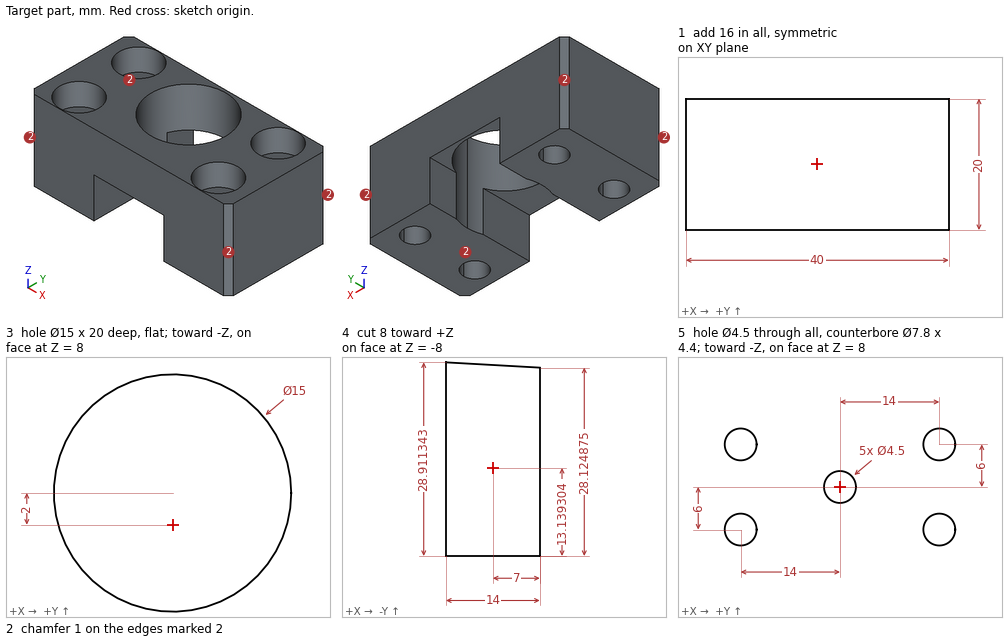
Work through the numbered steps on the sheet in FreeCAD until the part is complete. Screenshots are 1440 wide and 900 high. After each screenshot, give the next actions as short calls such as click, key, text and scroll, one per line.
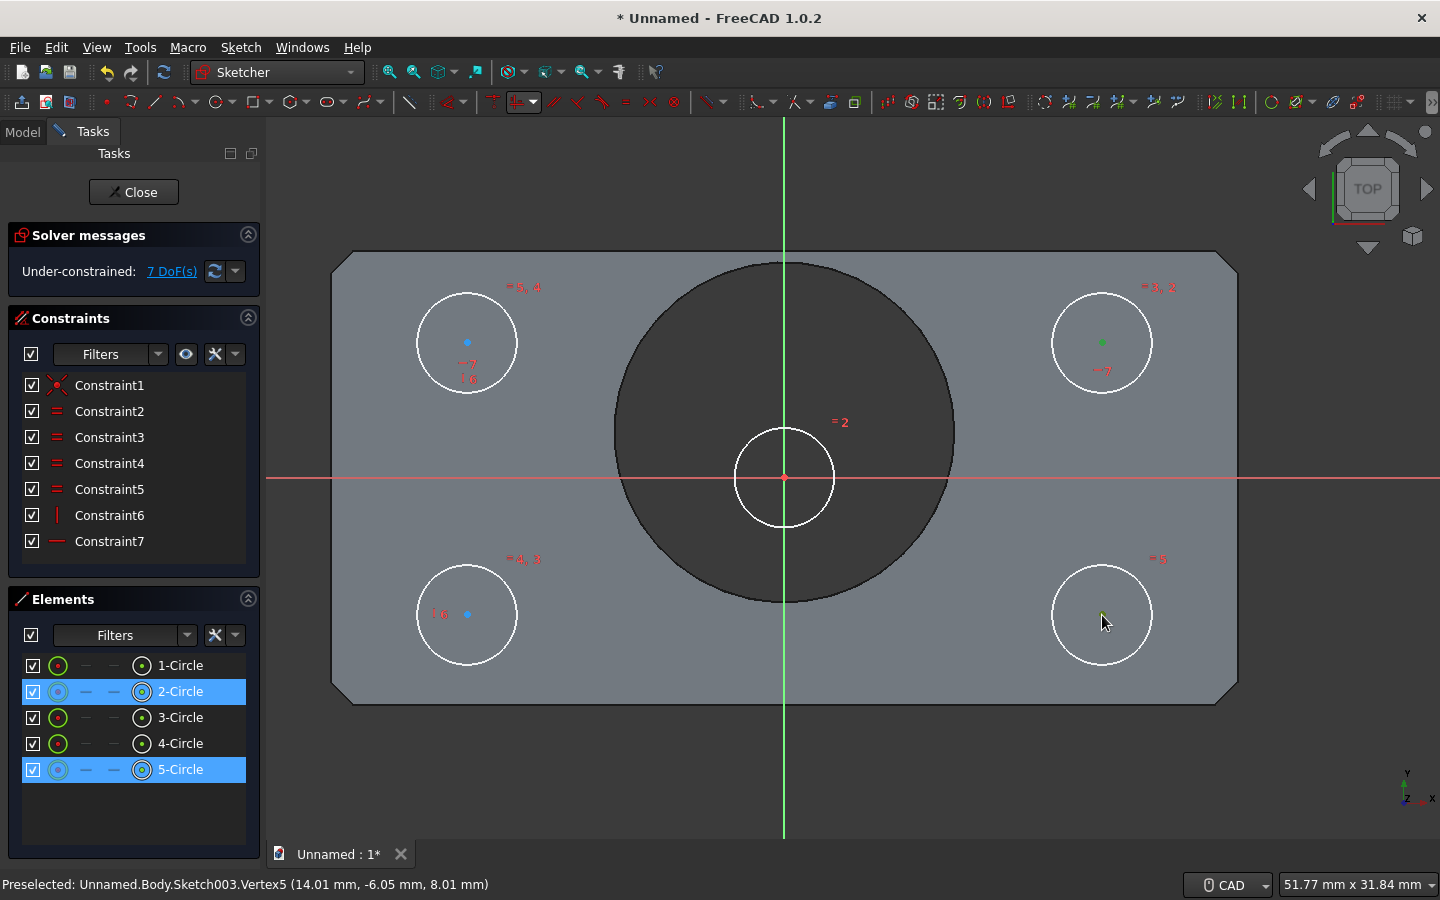
key(v)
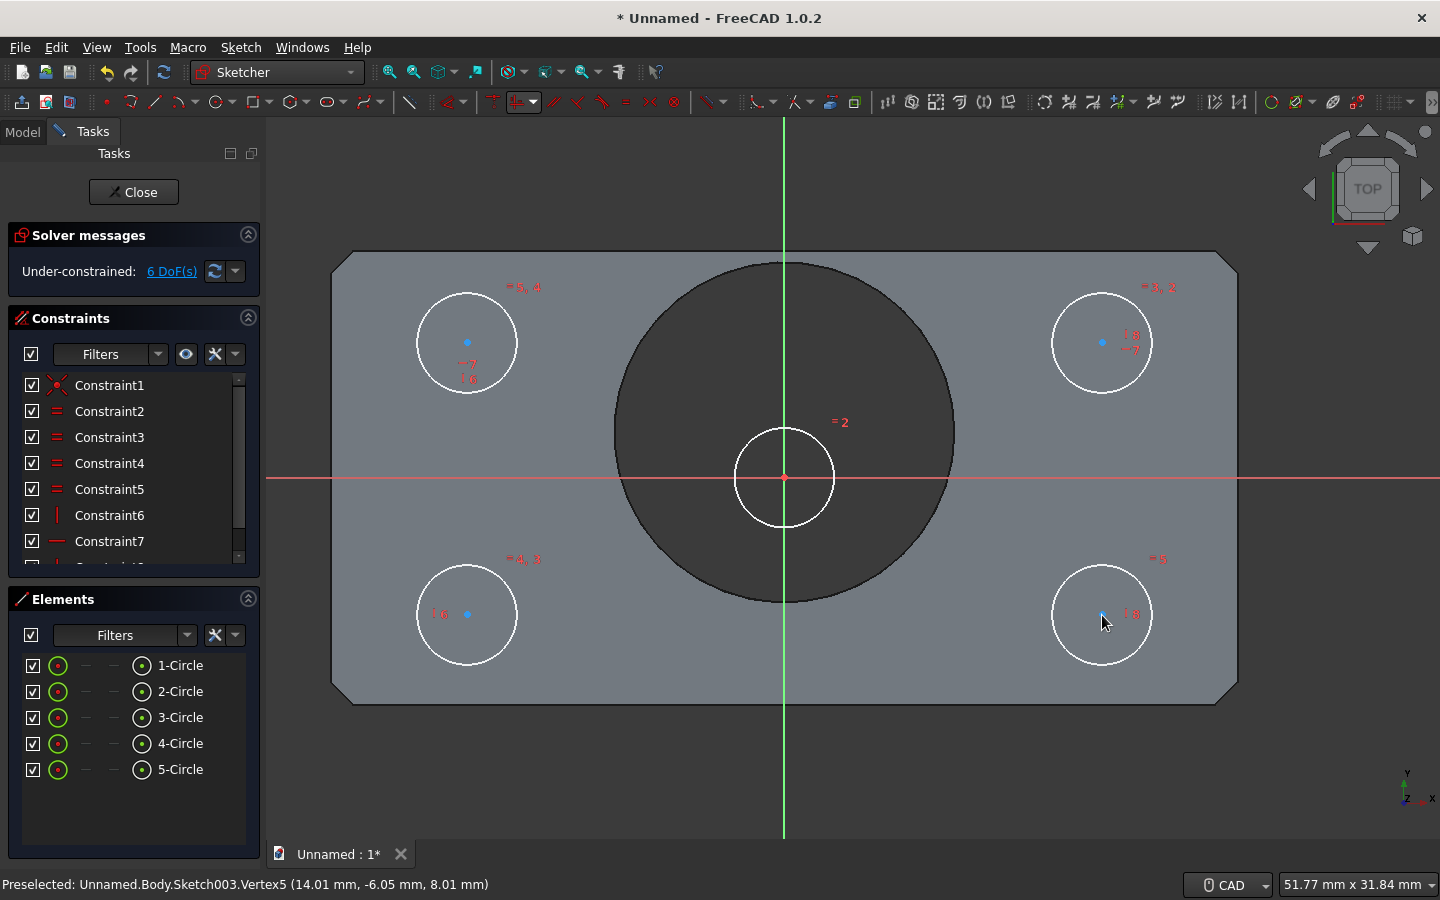
click(467, 615)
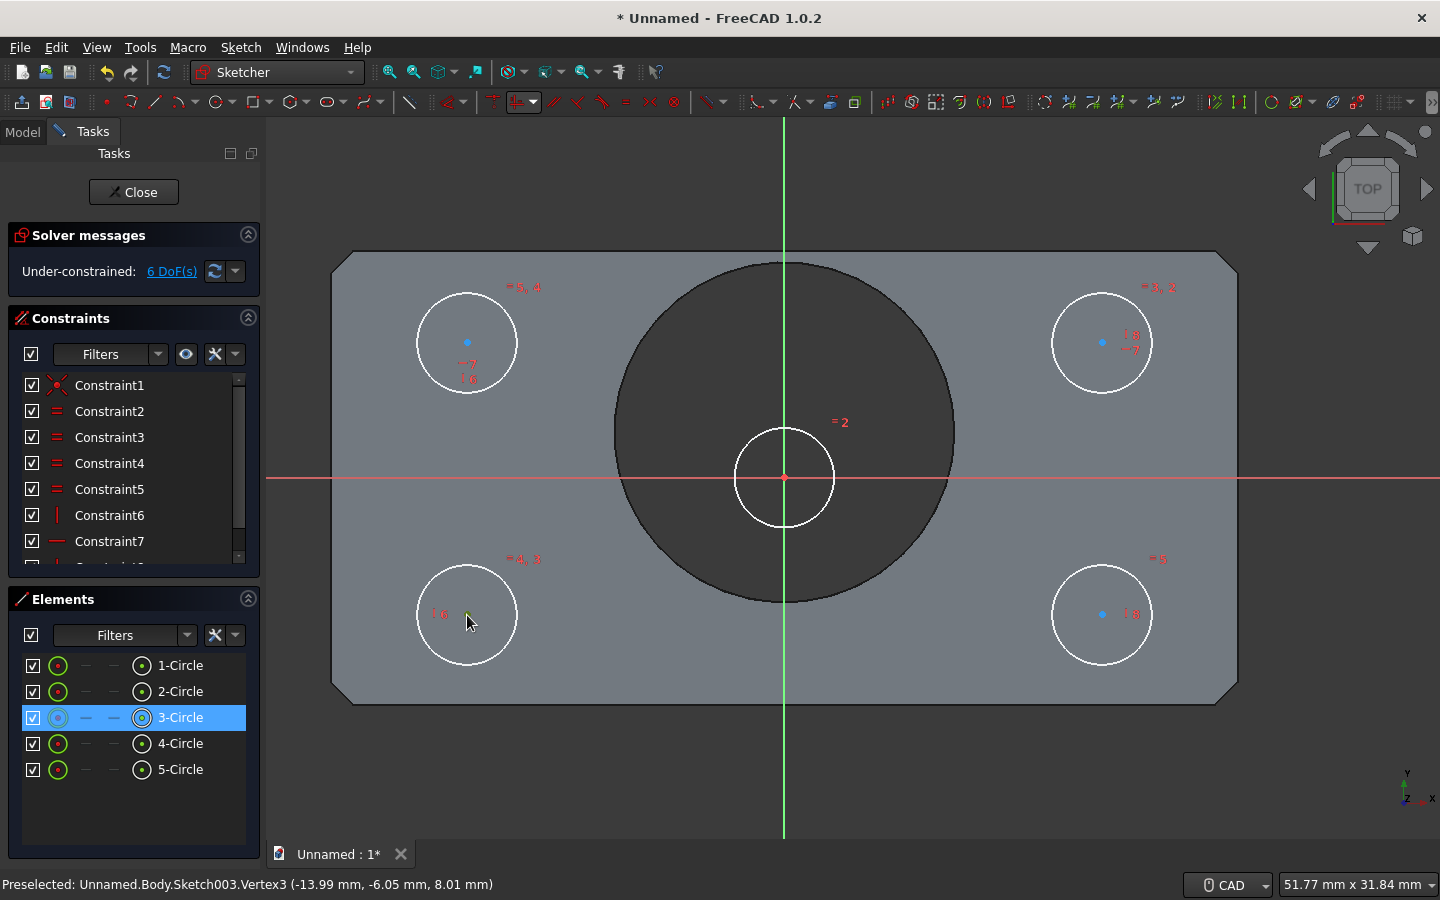
click(1102, 615)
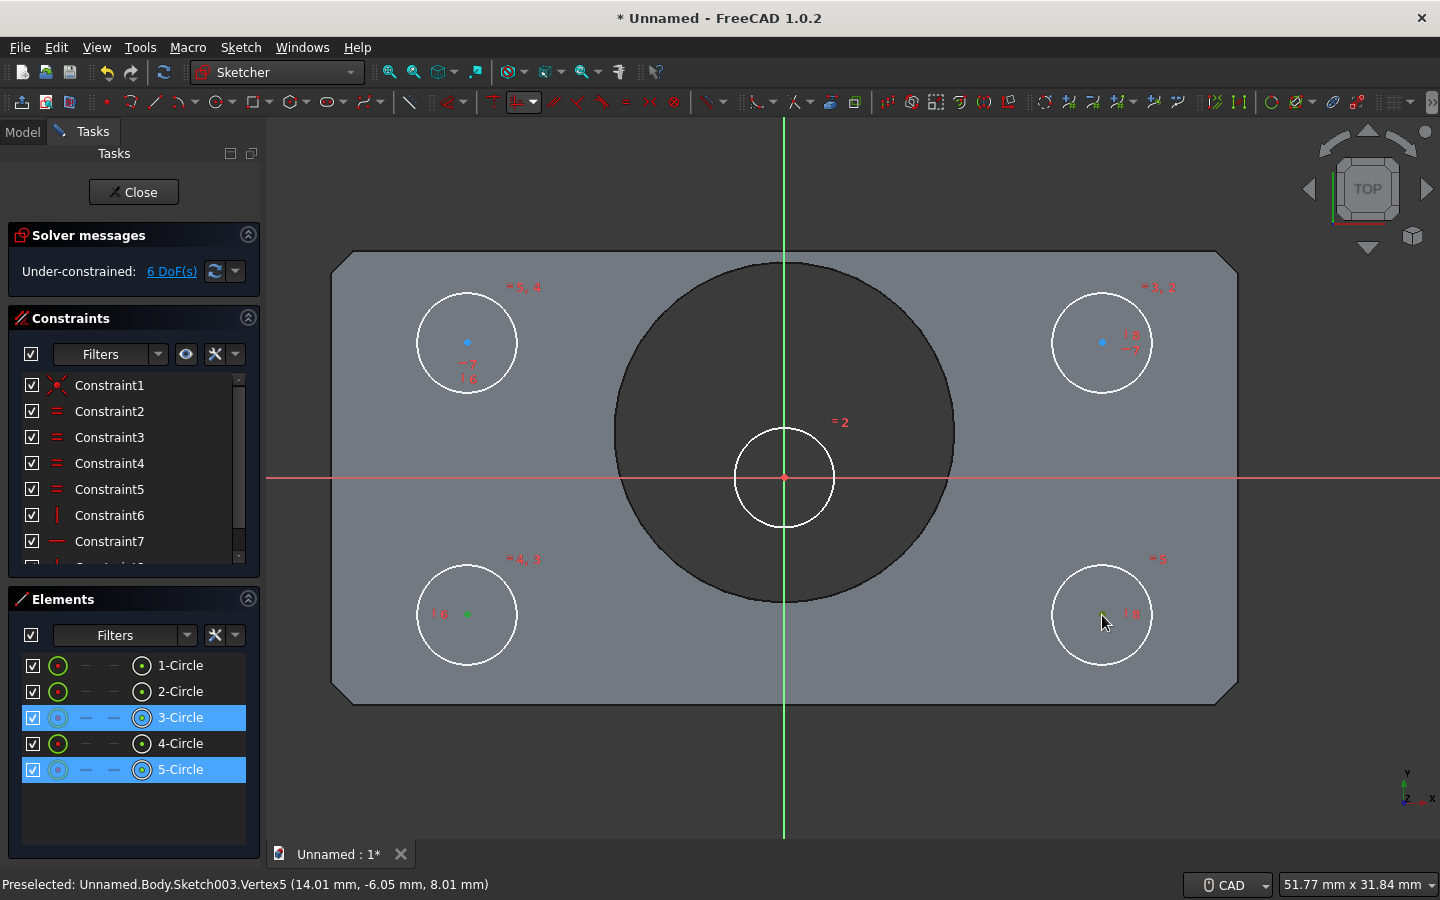
key(h)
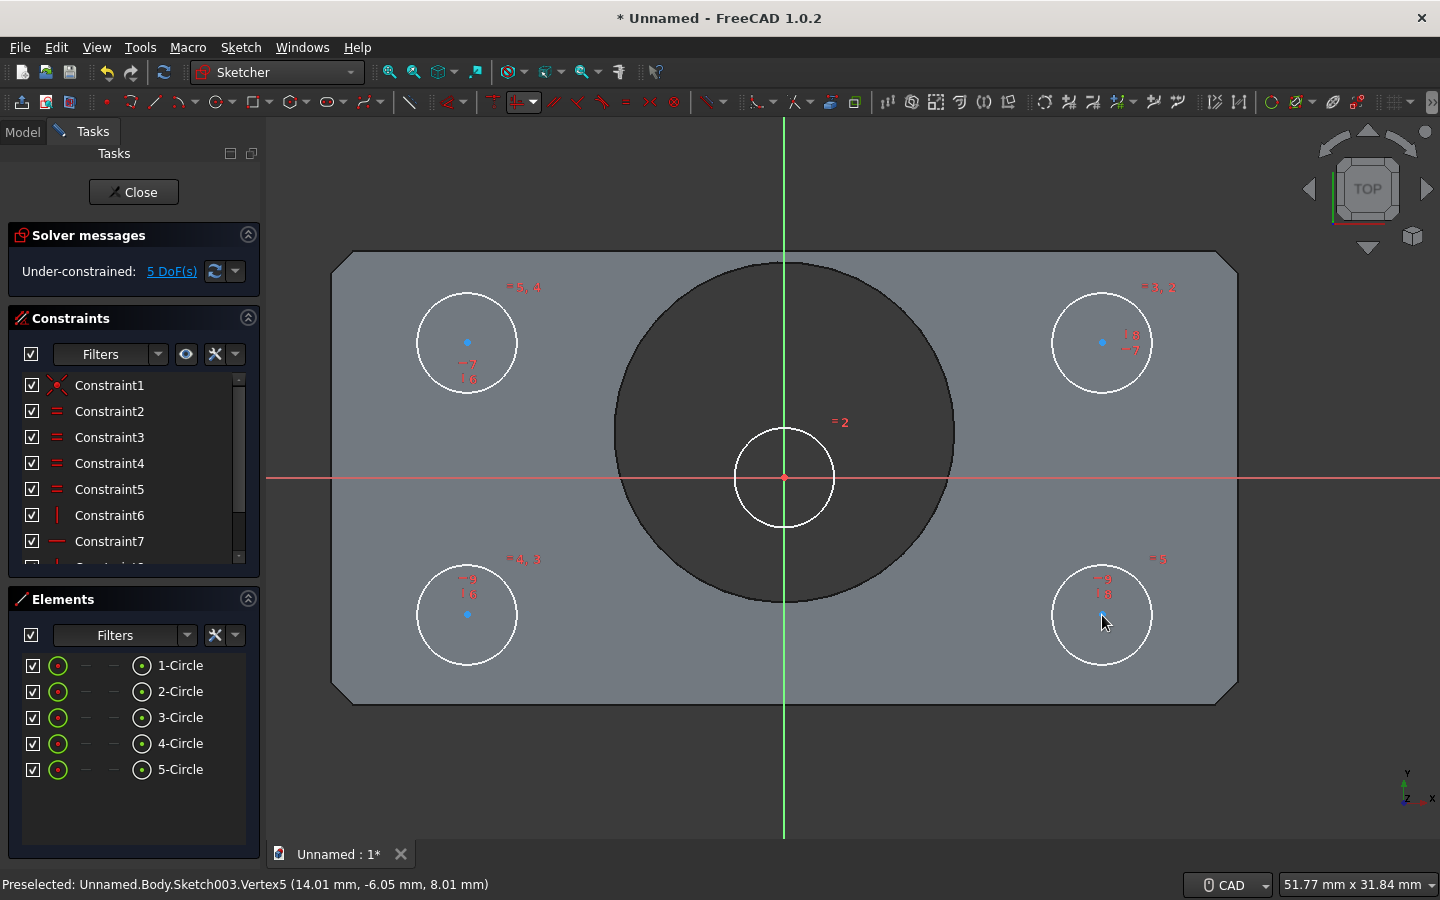
key(d)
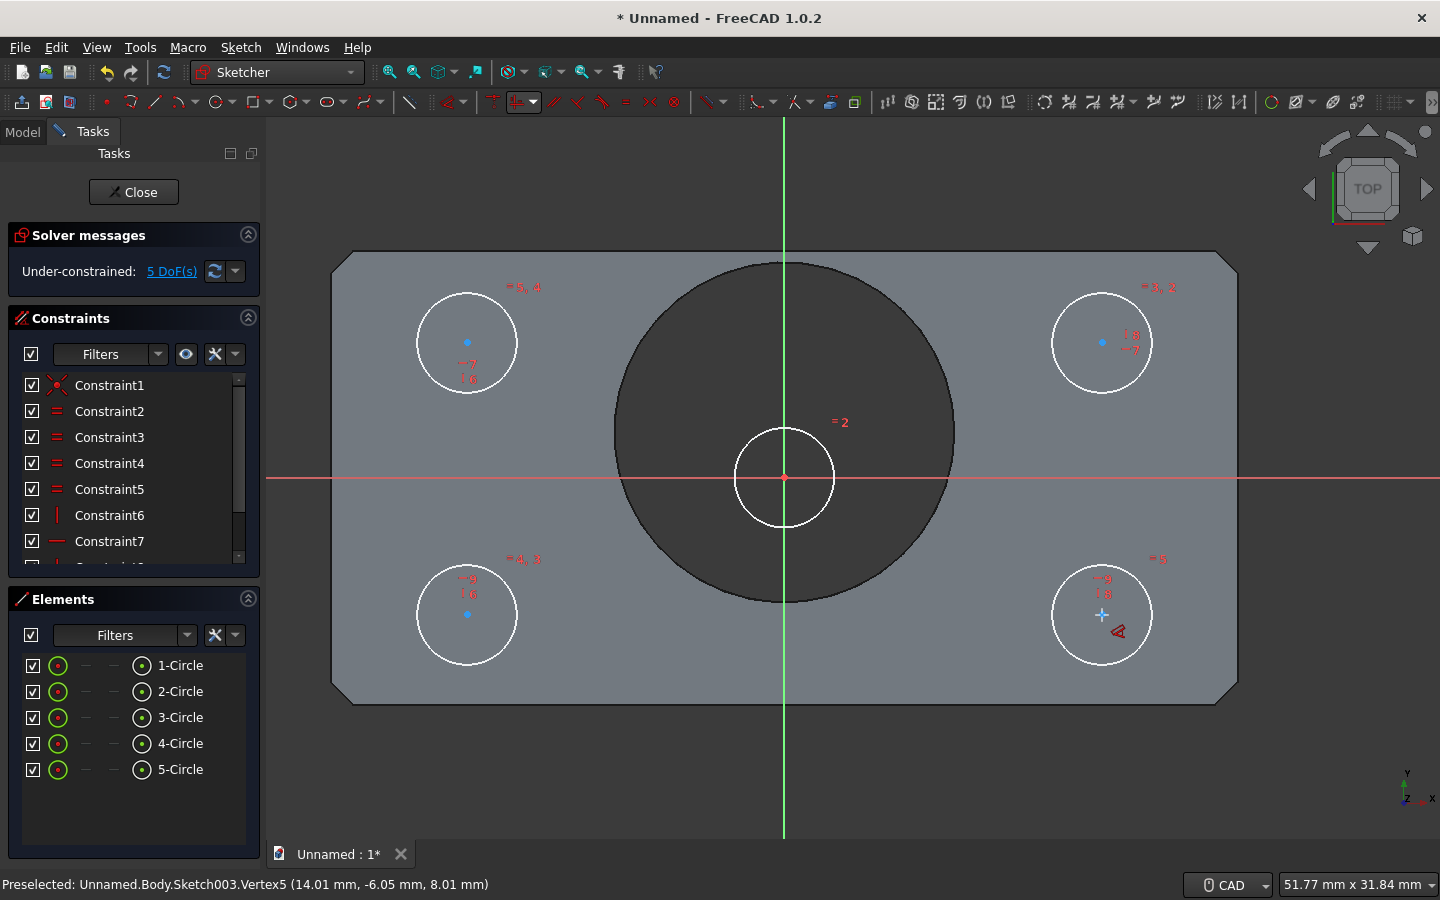
click(819, 442)
click(841, 419)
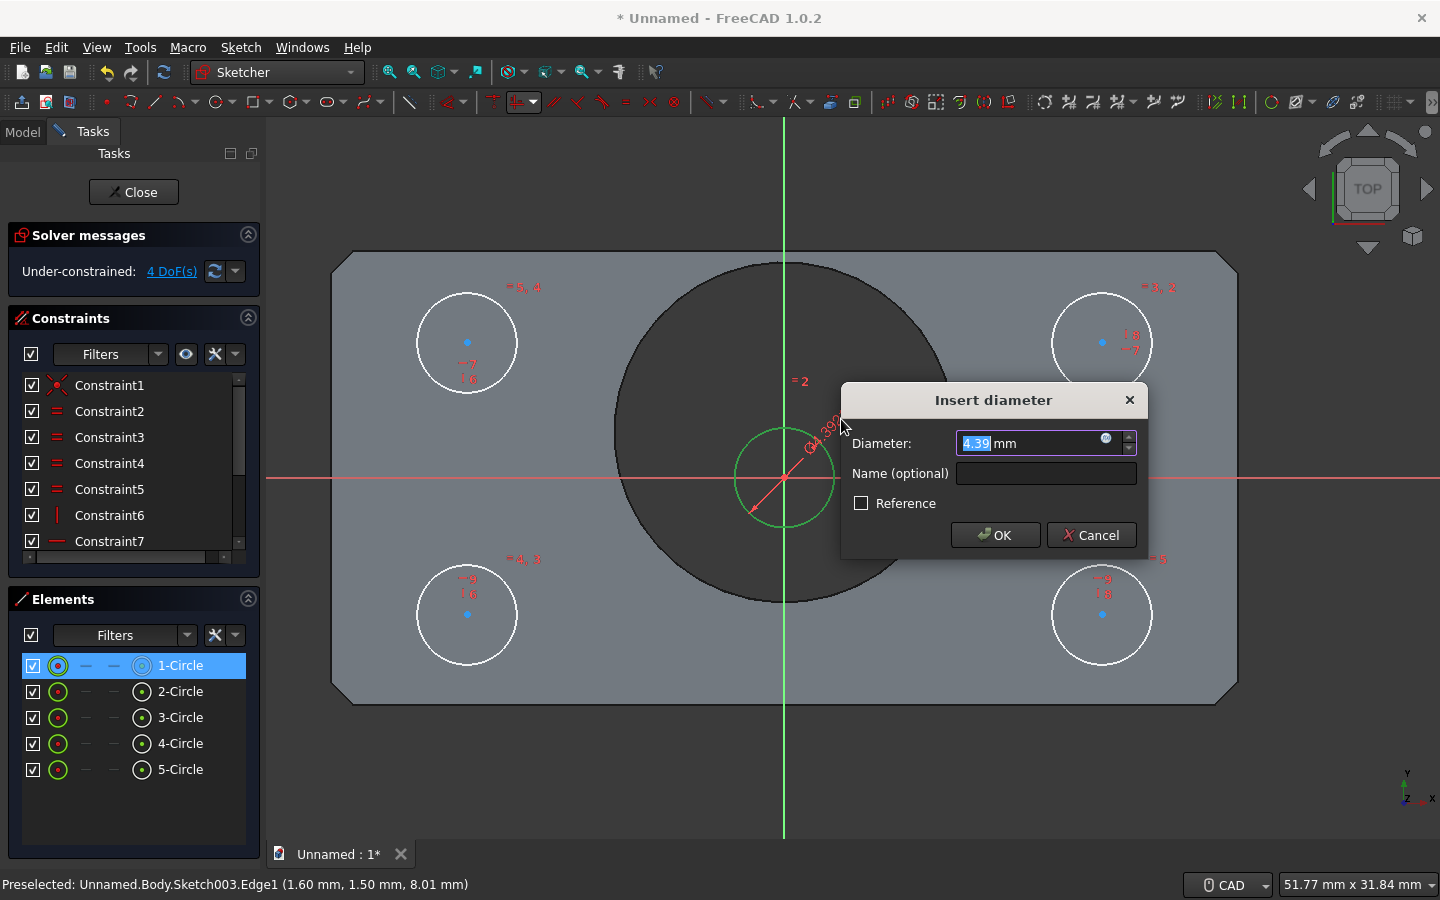
text(4.5)
key(Return)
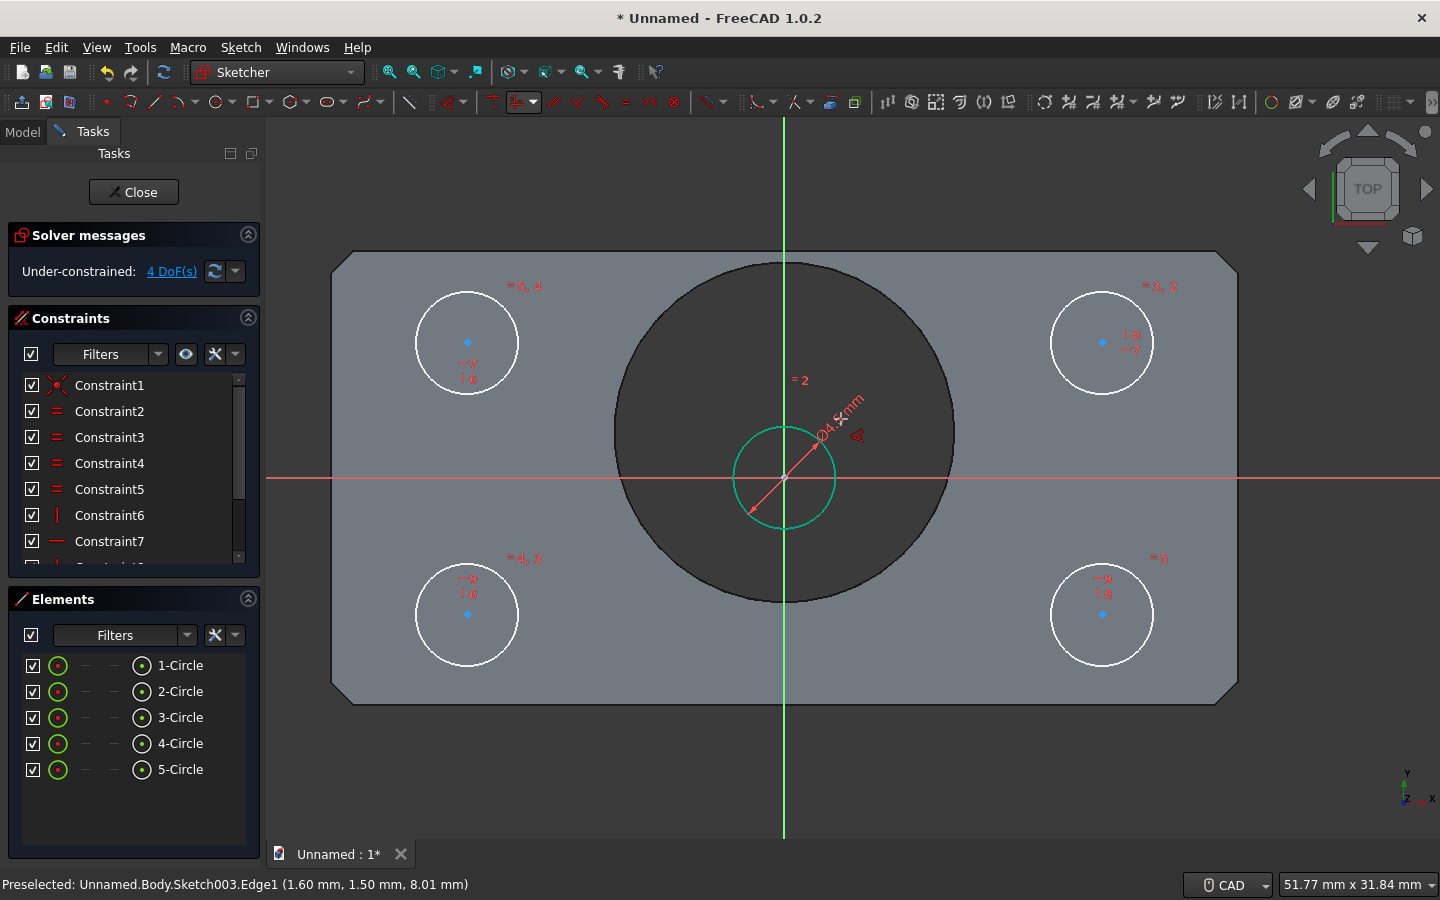
click(1102, 343)
click(1136, 410)